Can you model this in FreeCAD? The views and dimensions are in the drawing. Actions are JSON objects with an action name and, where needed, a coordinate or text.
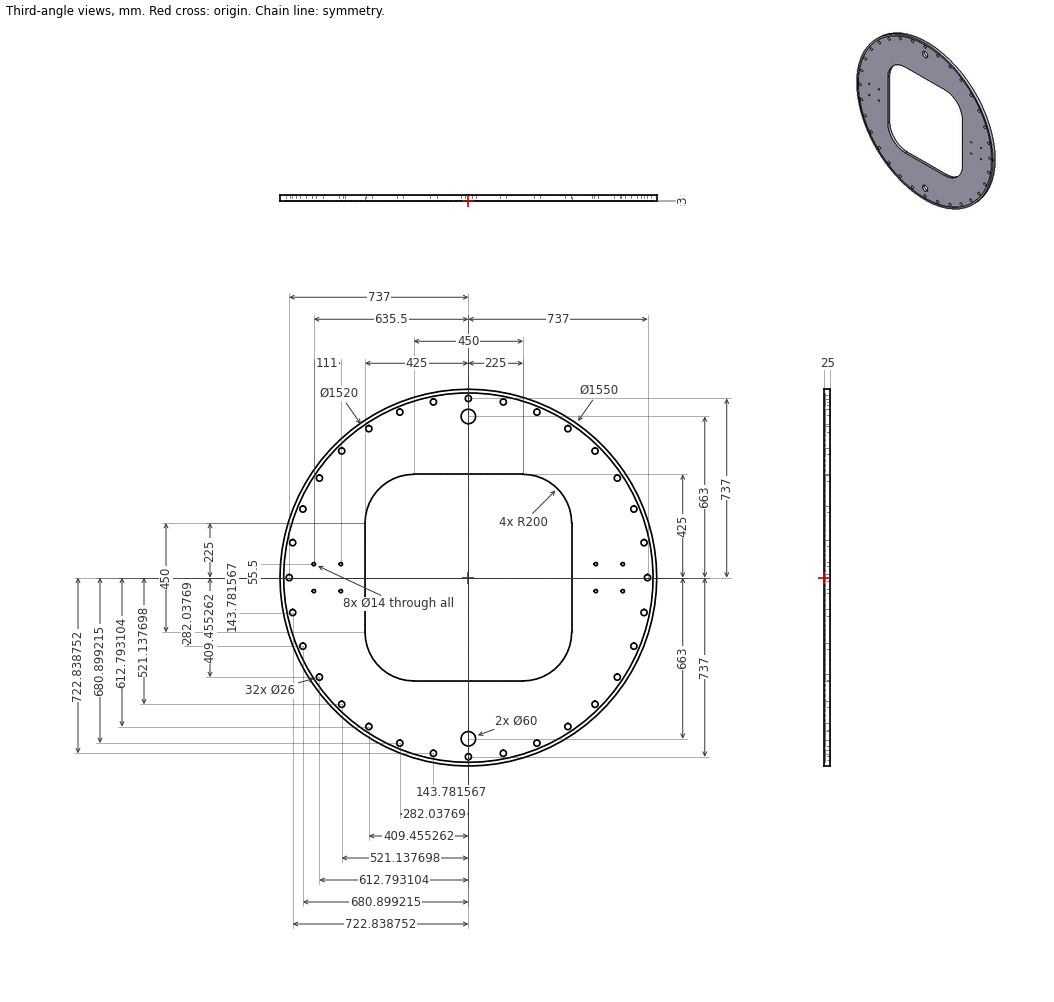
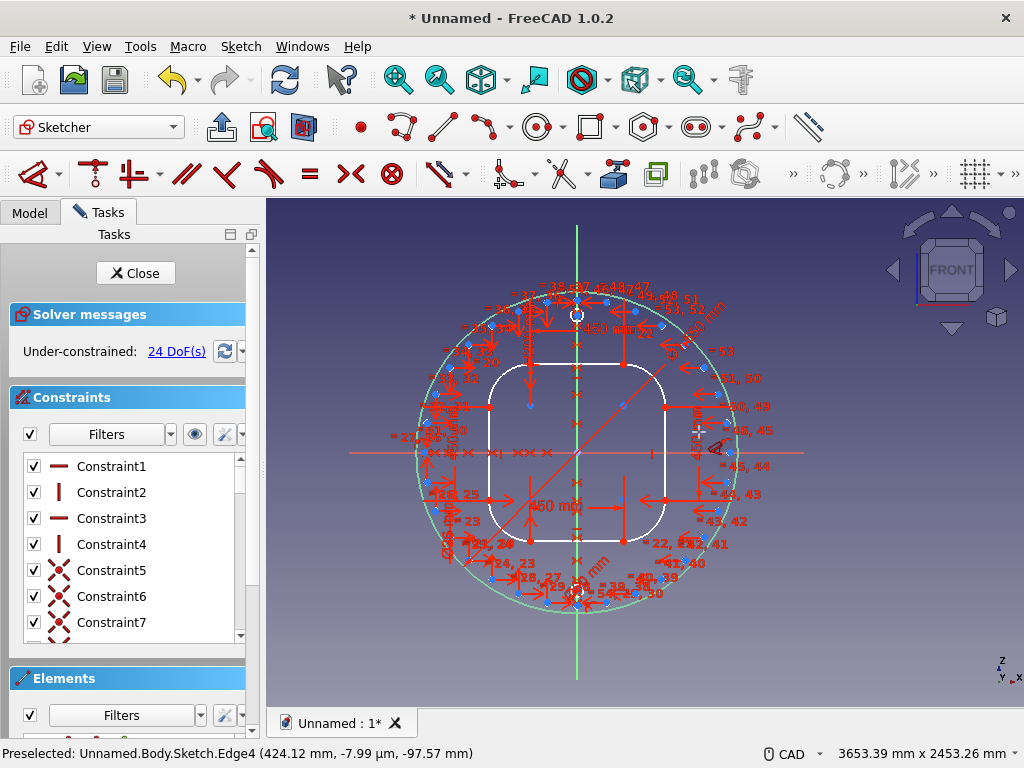
{"action": "left_click", "coordinate": [577, 606]}
{"action": "left_click", "coordinate": [611, 476]}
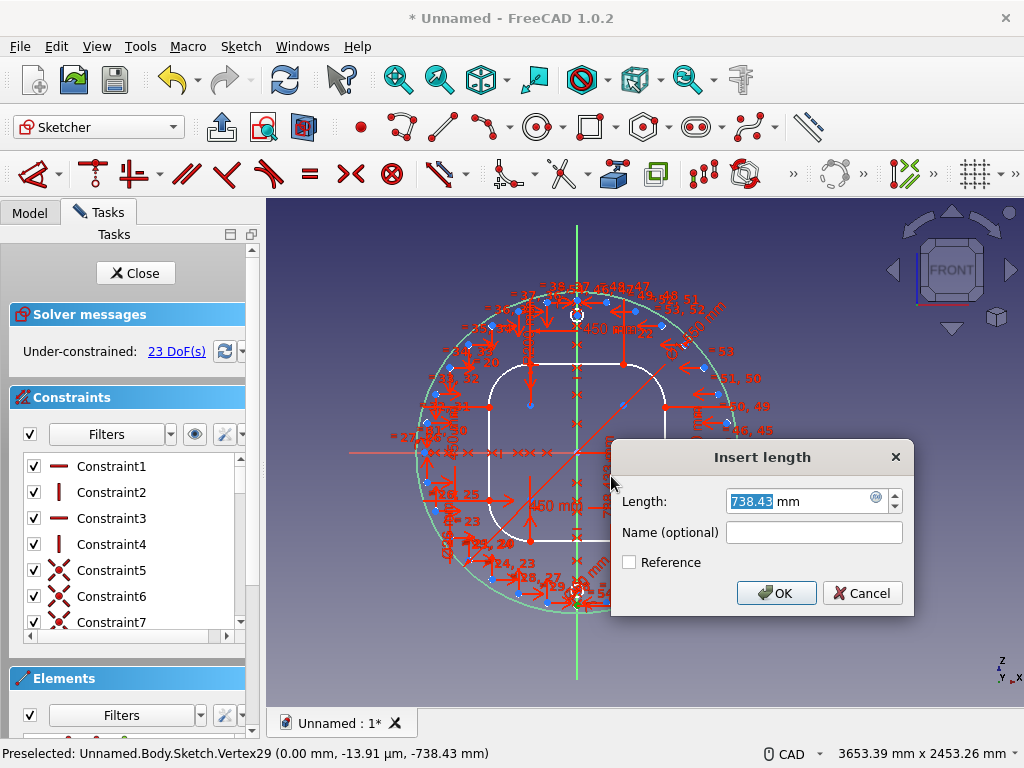
{"action": "type", "text": "737"}
{"action": "key", "text": "Return"}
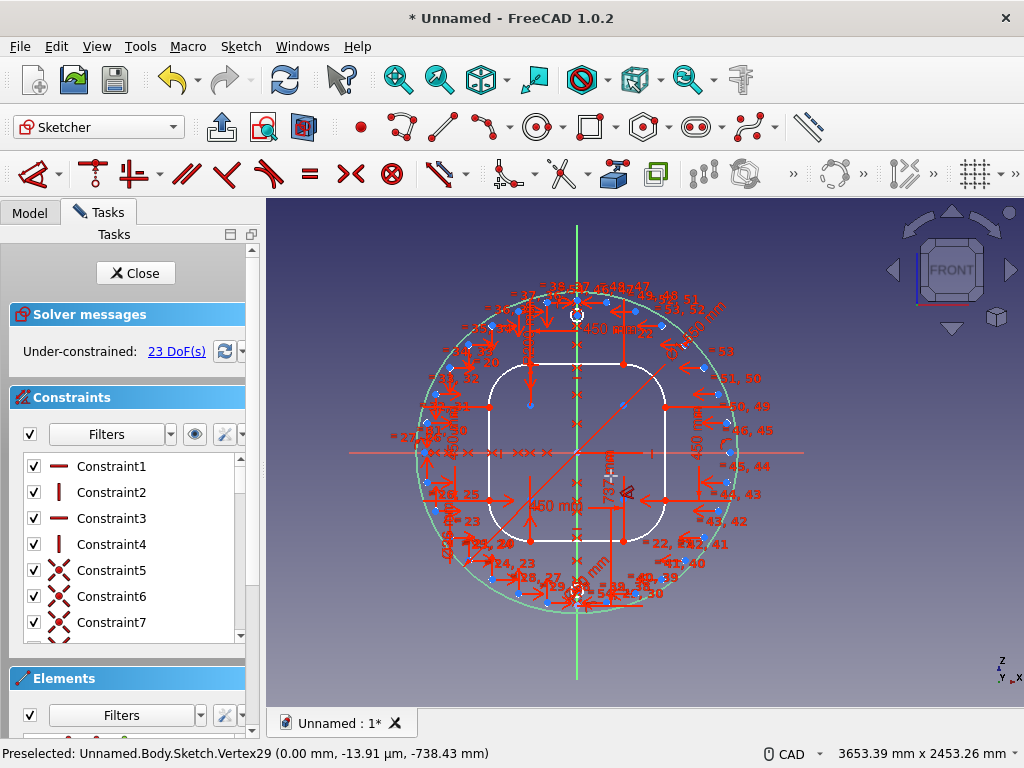
{"action": "left_click", "coordinate": [577, 591]}
{"action": "left_click", "coordinate": [635, 522]}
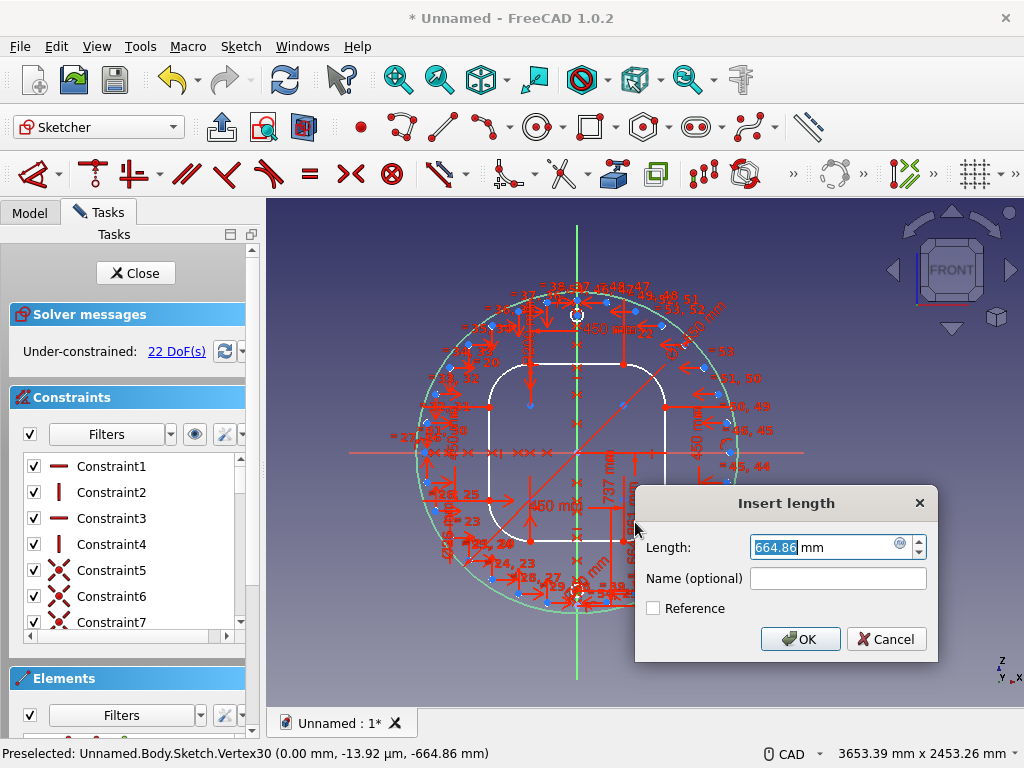
{"action": "type", "text": "663"}
{"action": "key", "text": "Return"}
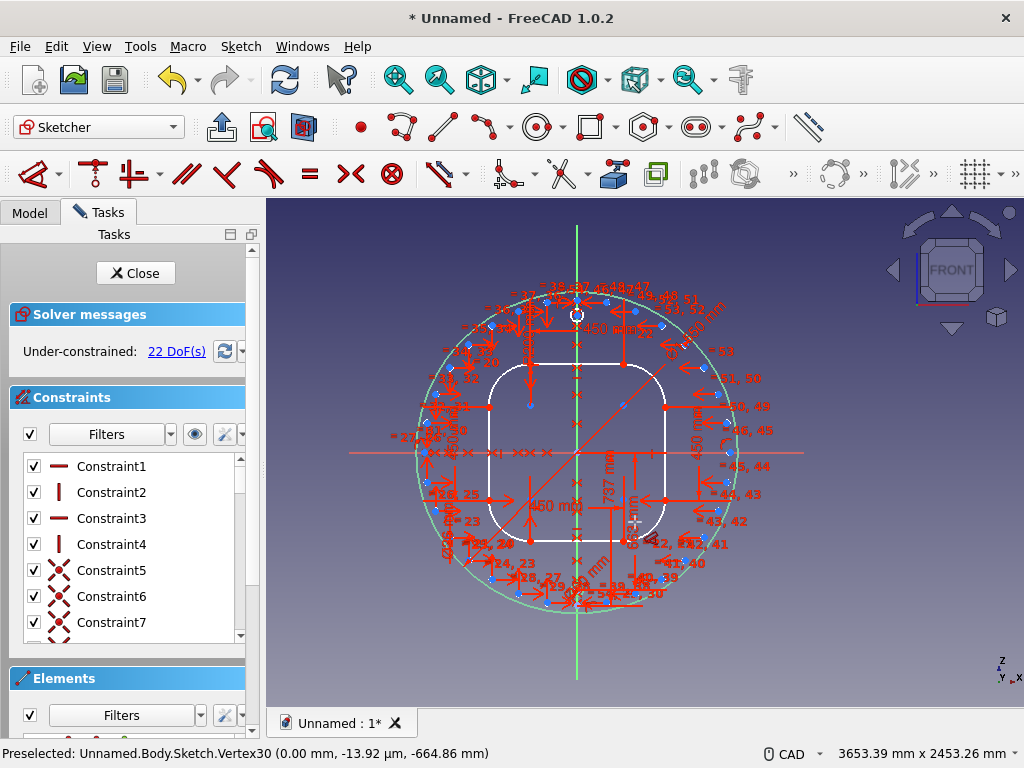
{"action": "left_click", "coordinate": [424, 453]}
{"action": "left_click", "coordinate": [465, 487]}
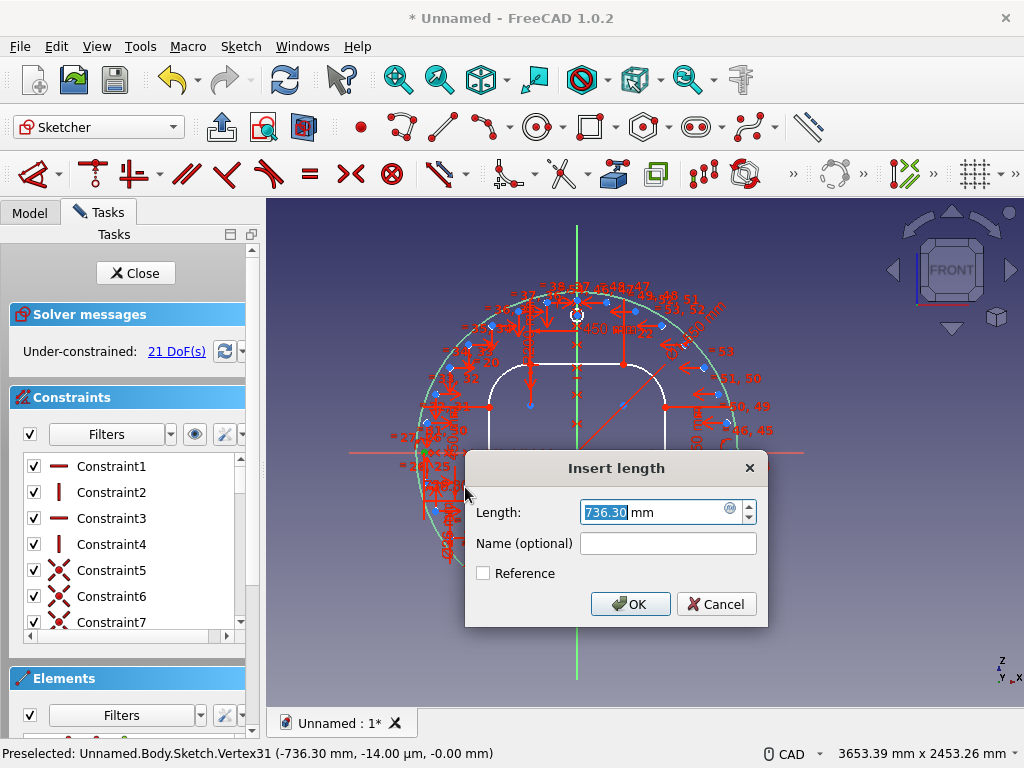
{"action": "type", "text": "737"}
{"action": "key", "text": "Return"}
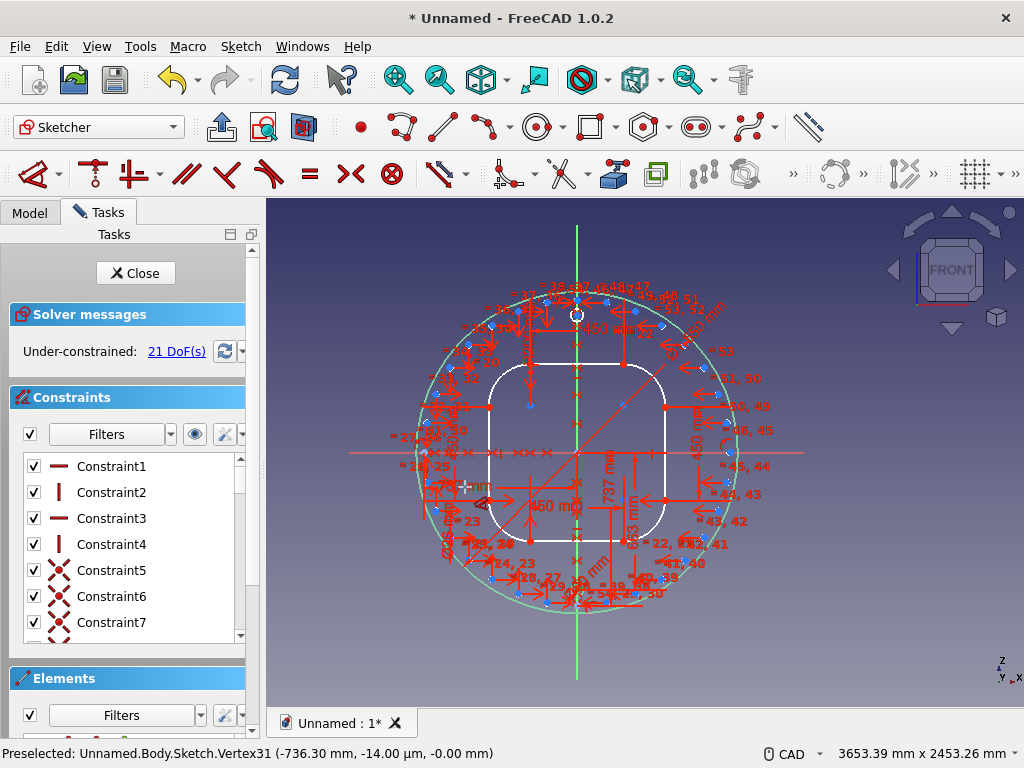
{"action": "left_click", "coordinate": [730, 453]}
{"action": "left_click", "coordinate": [689, 487]}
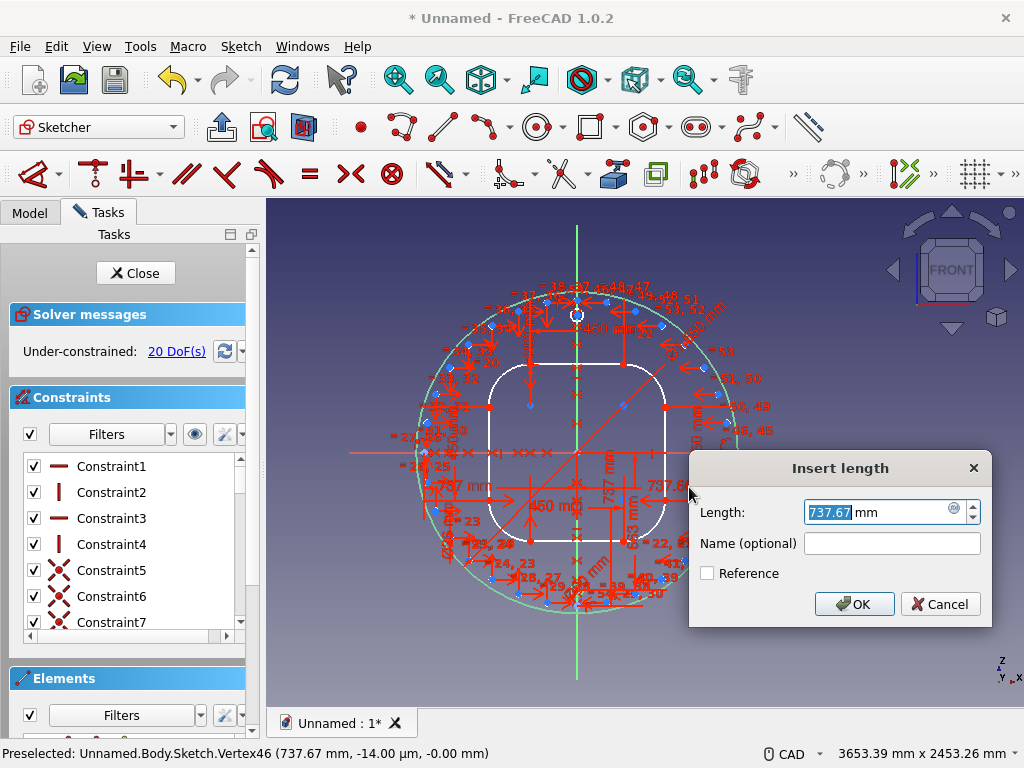
{"action": "type", "text": "737"}
{"action": "key", "text": "Return"}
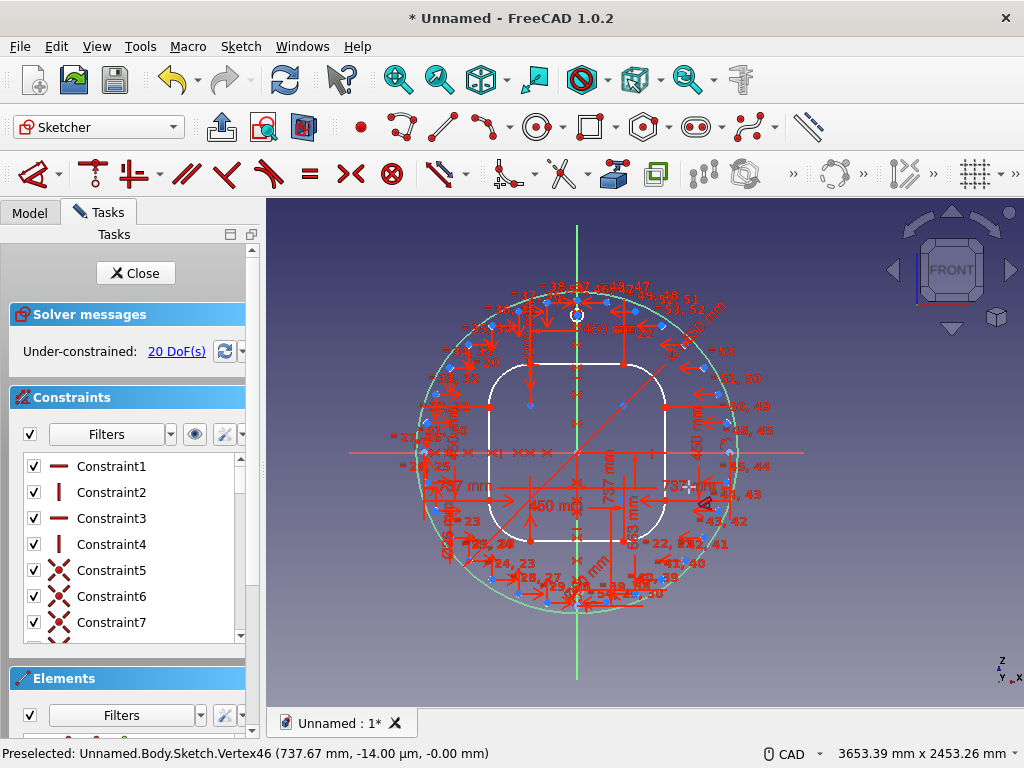
{"action": "left_click", "coordinate": [577, 315]}
{"action": "left_click", "coordinate": [611, 384]}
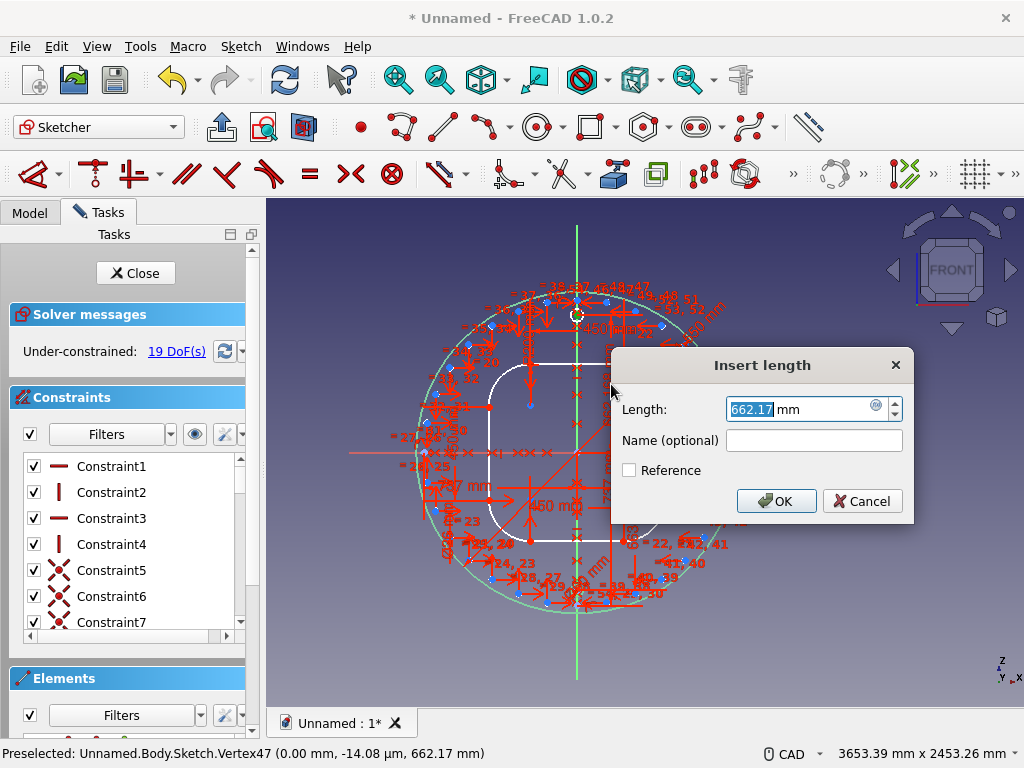
{"action": "type", "text": "663"}
{"action": "key", "text": "Return"}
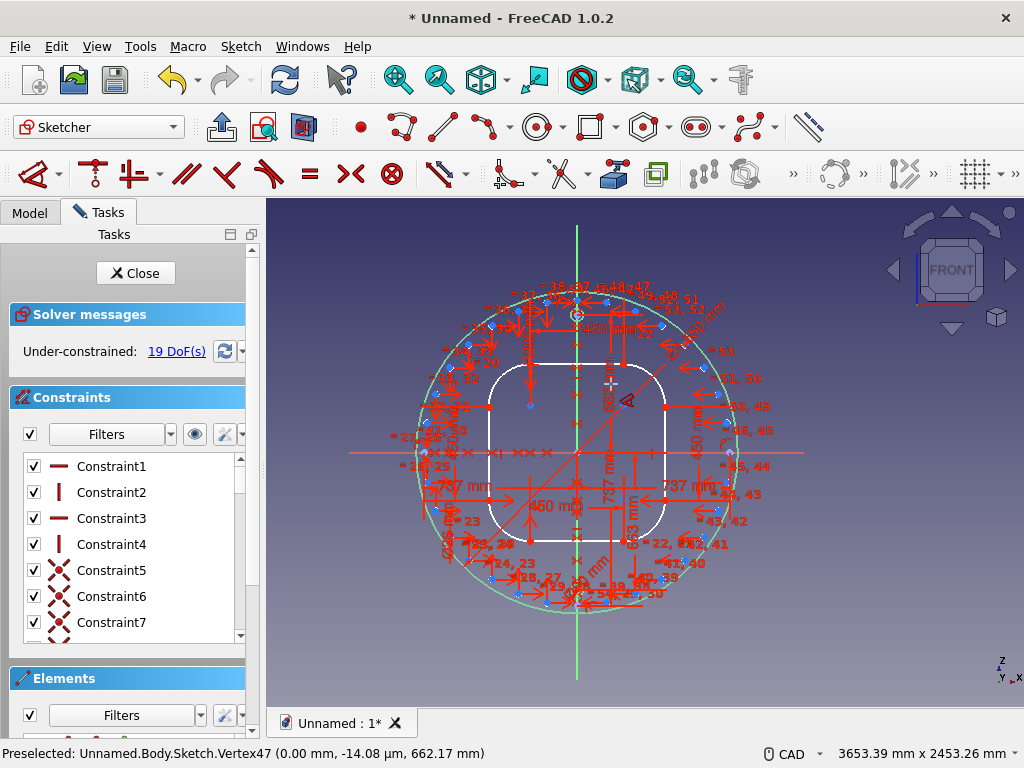
{"action": "left_click", "coordinate": [577, 300]}
{"action": "left_click", "coordinate": [611, 412]}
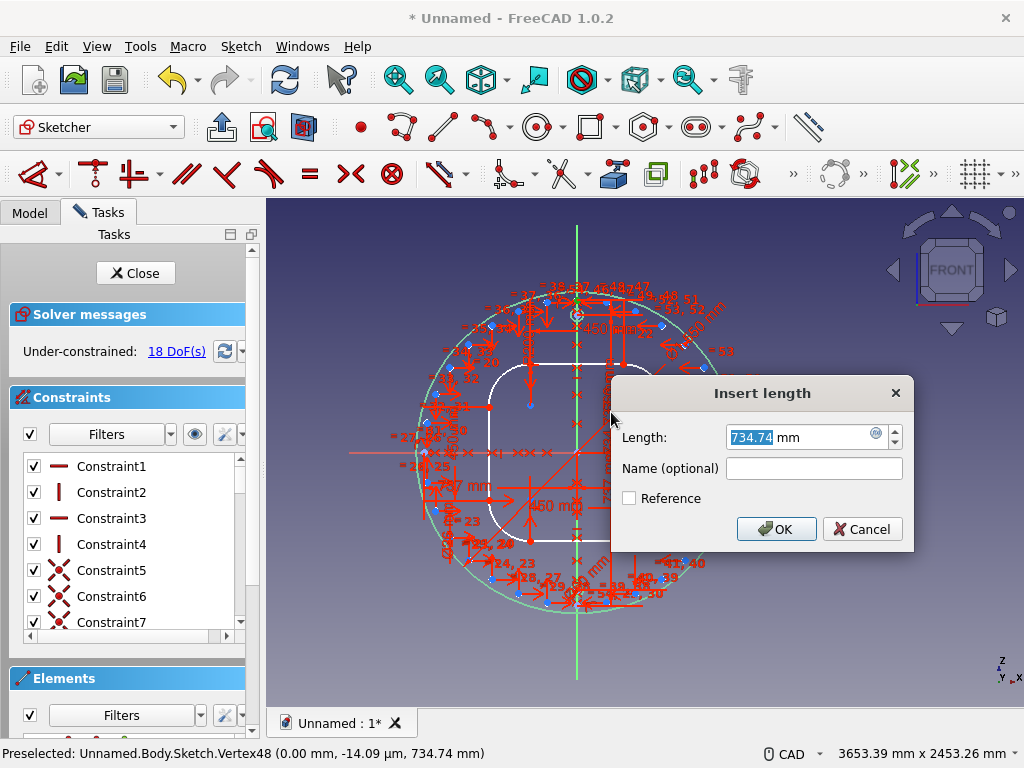
{"action": "type", "text": "737"}
{"action": "key", "text": "Return"}